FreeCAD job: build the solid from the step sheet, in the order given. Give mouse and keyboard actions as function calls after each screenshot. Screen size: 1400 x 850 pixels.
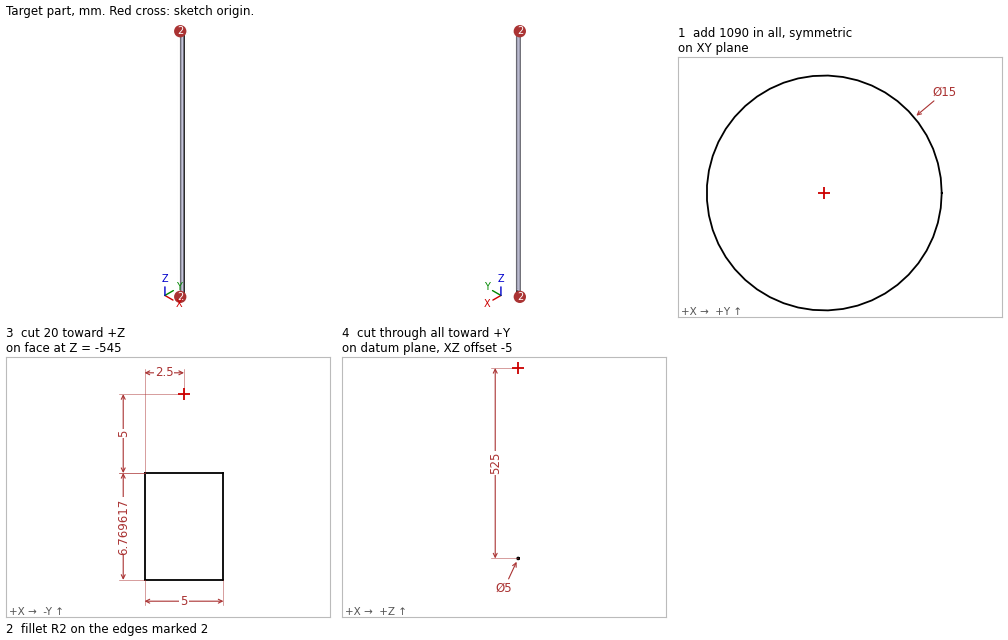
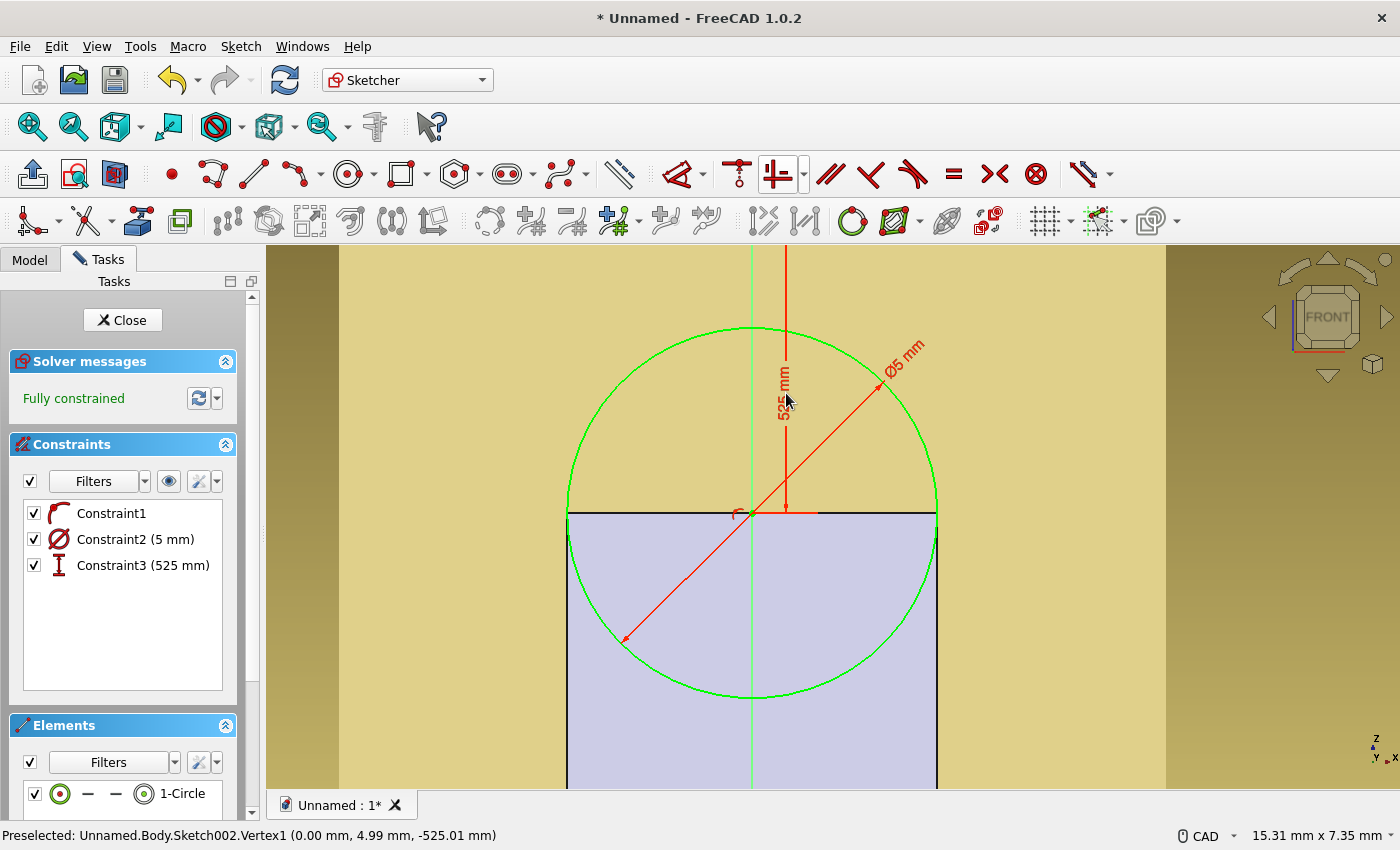
click(123, 320)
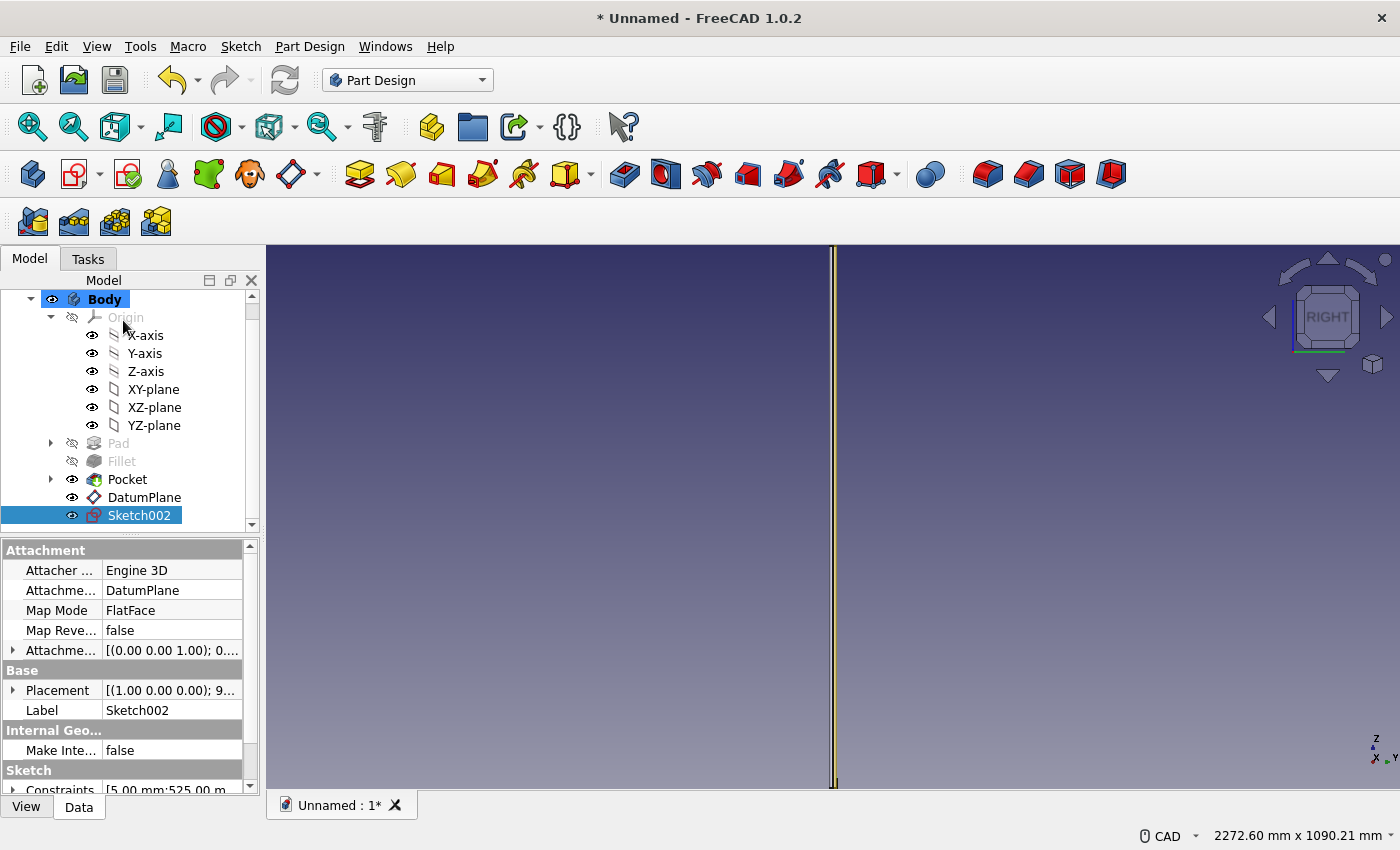
click(625, 174)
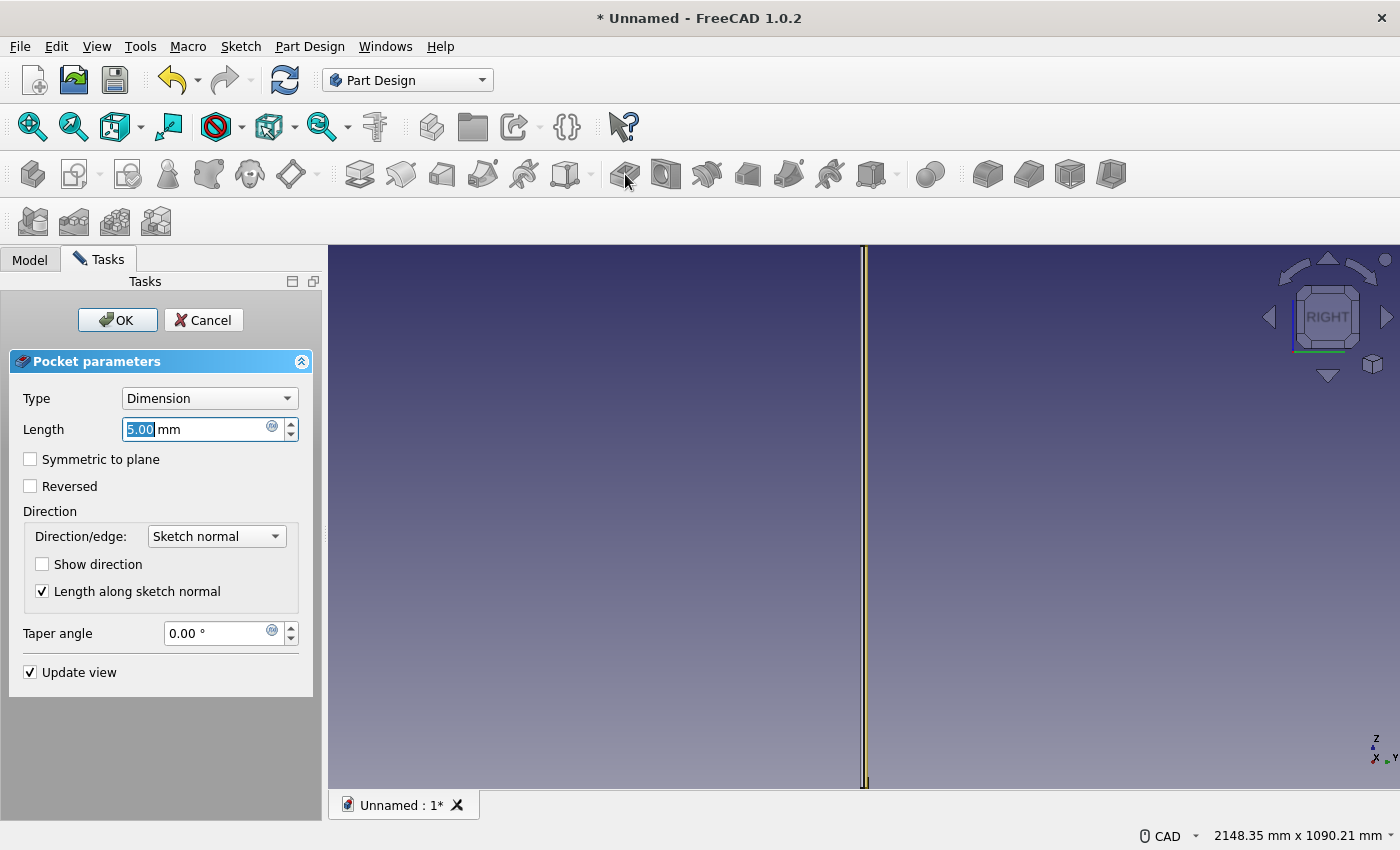
click(210, 398)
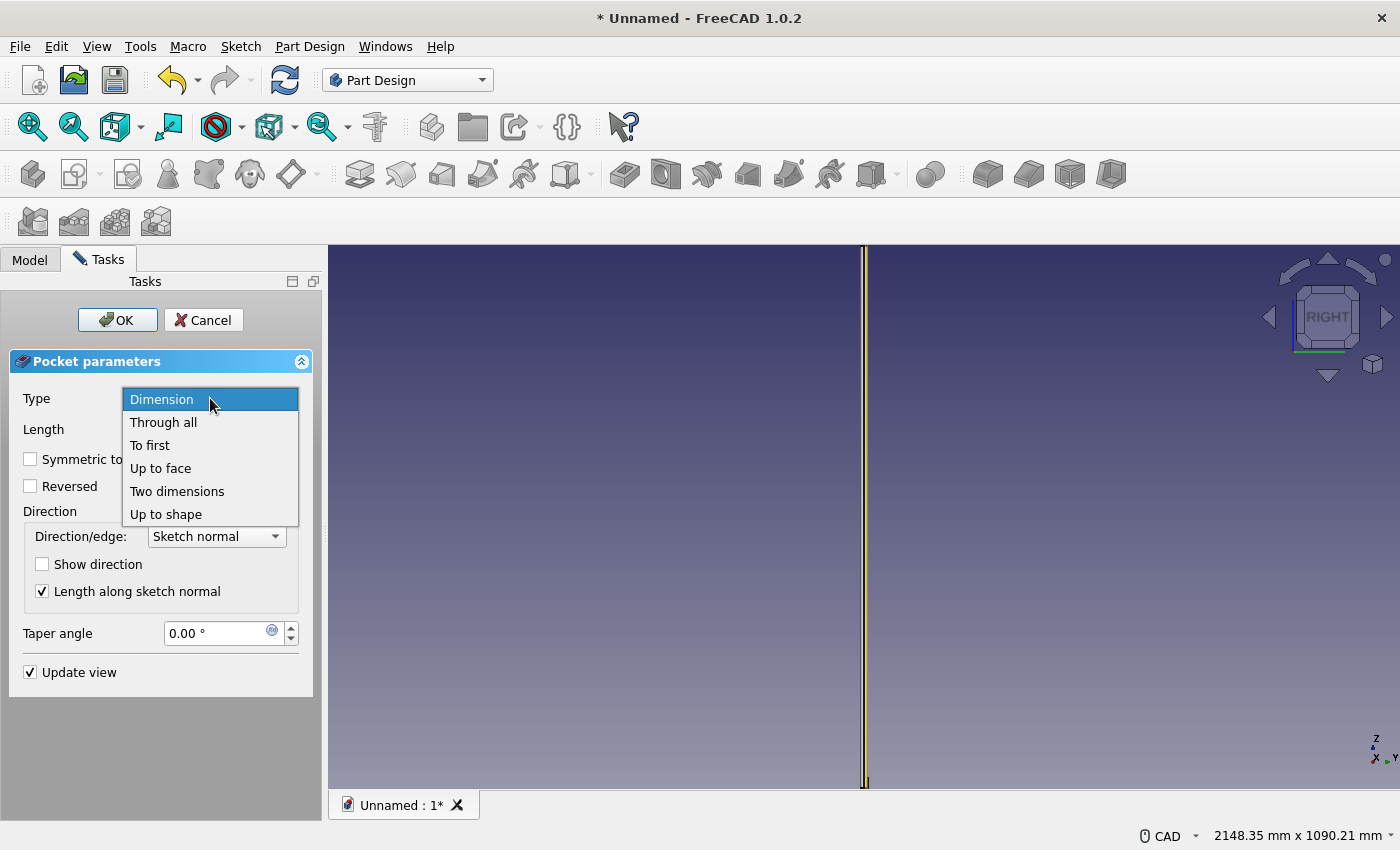
click(208, 422)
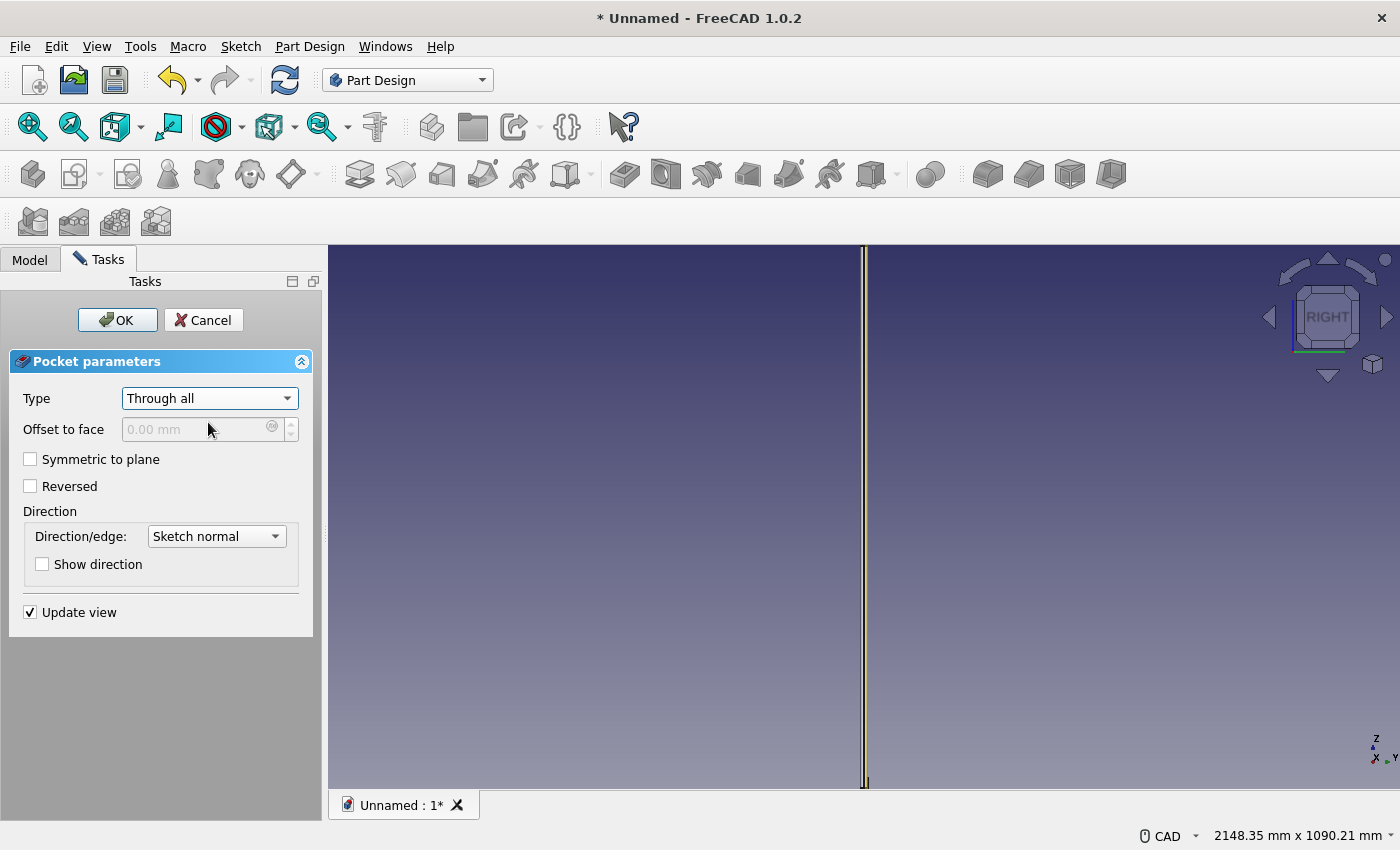
click(118, 320)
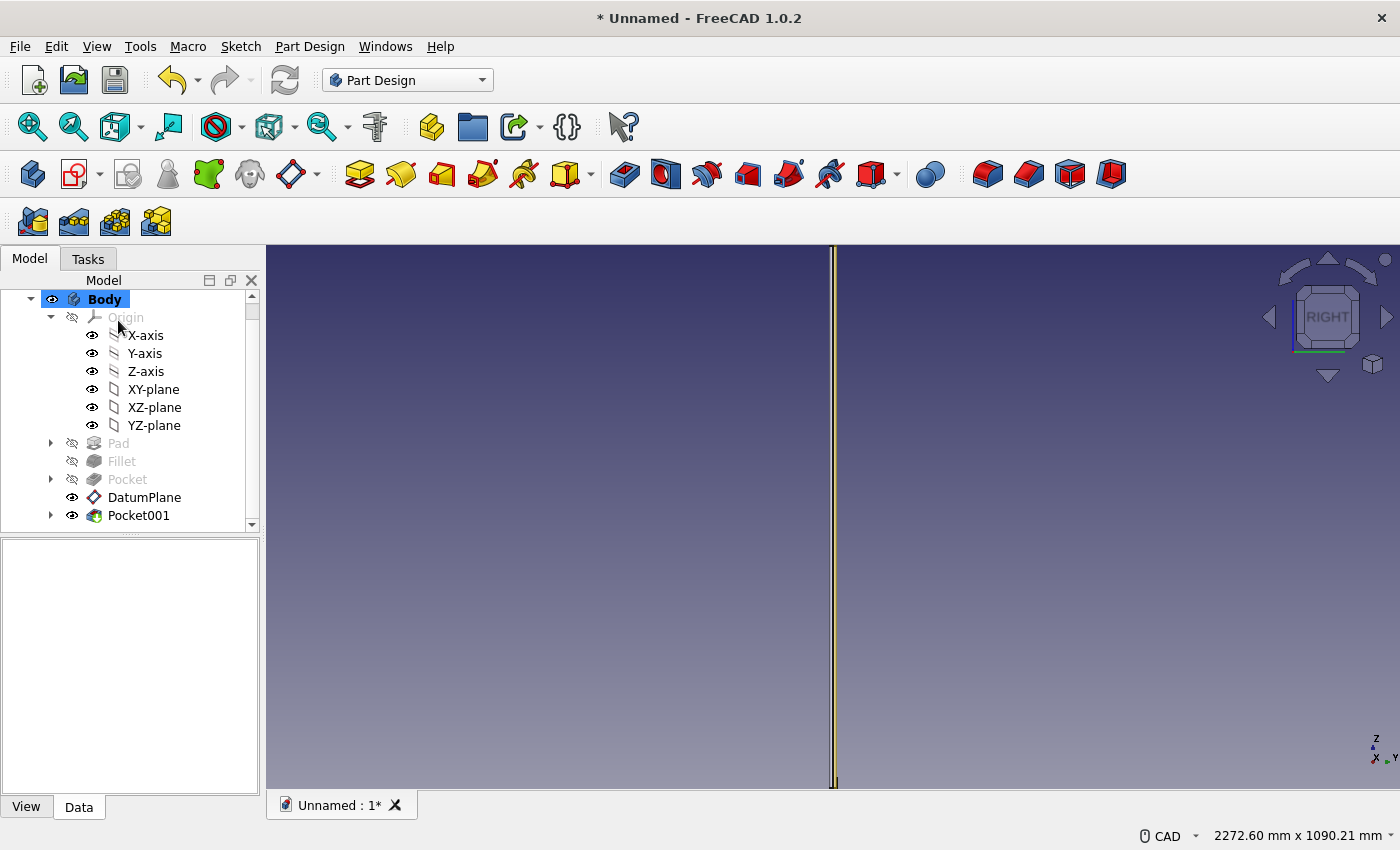
click(117, 497)
key(space)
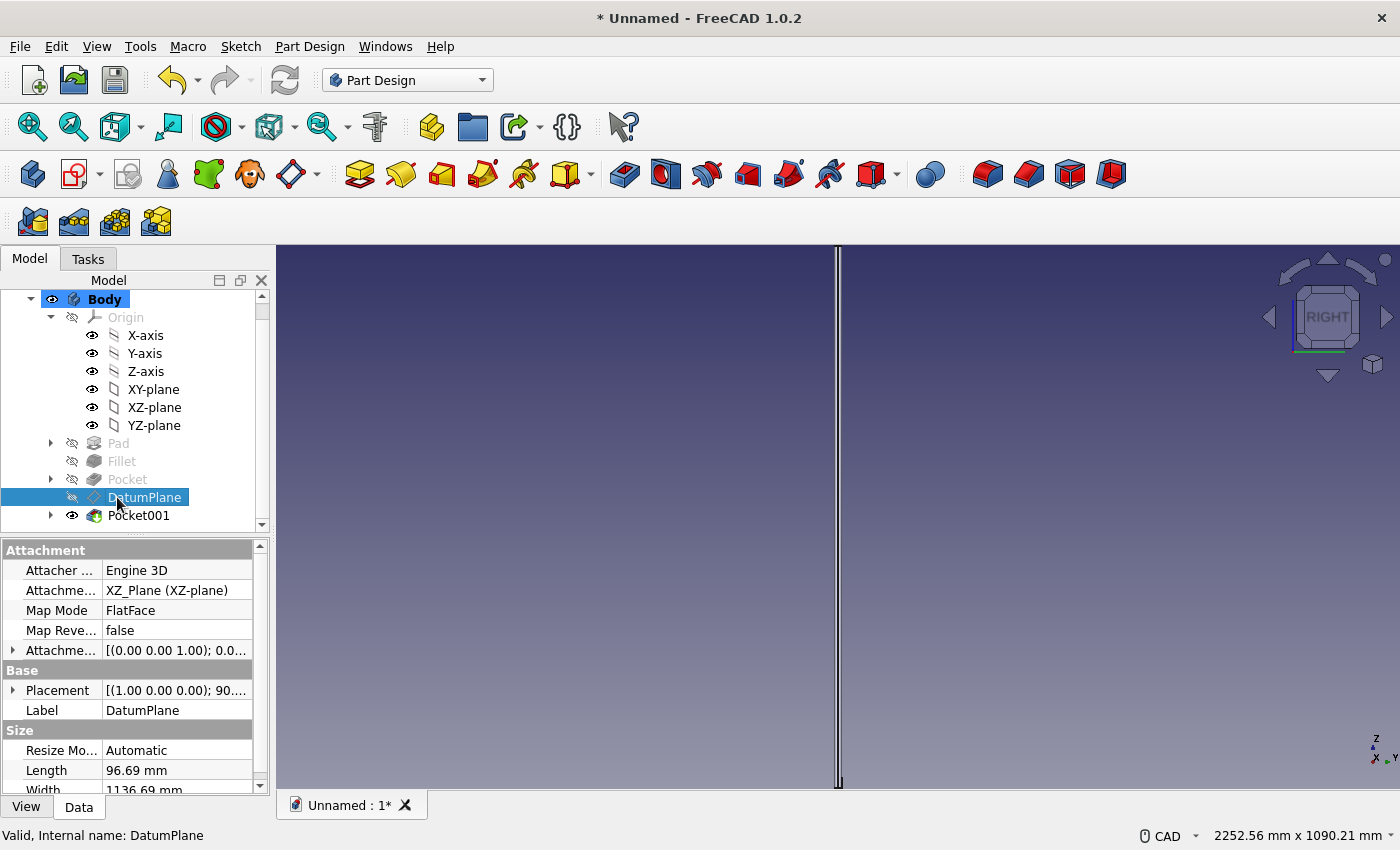
key(0)